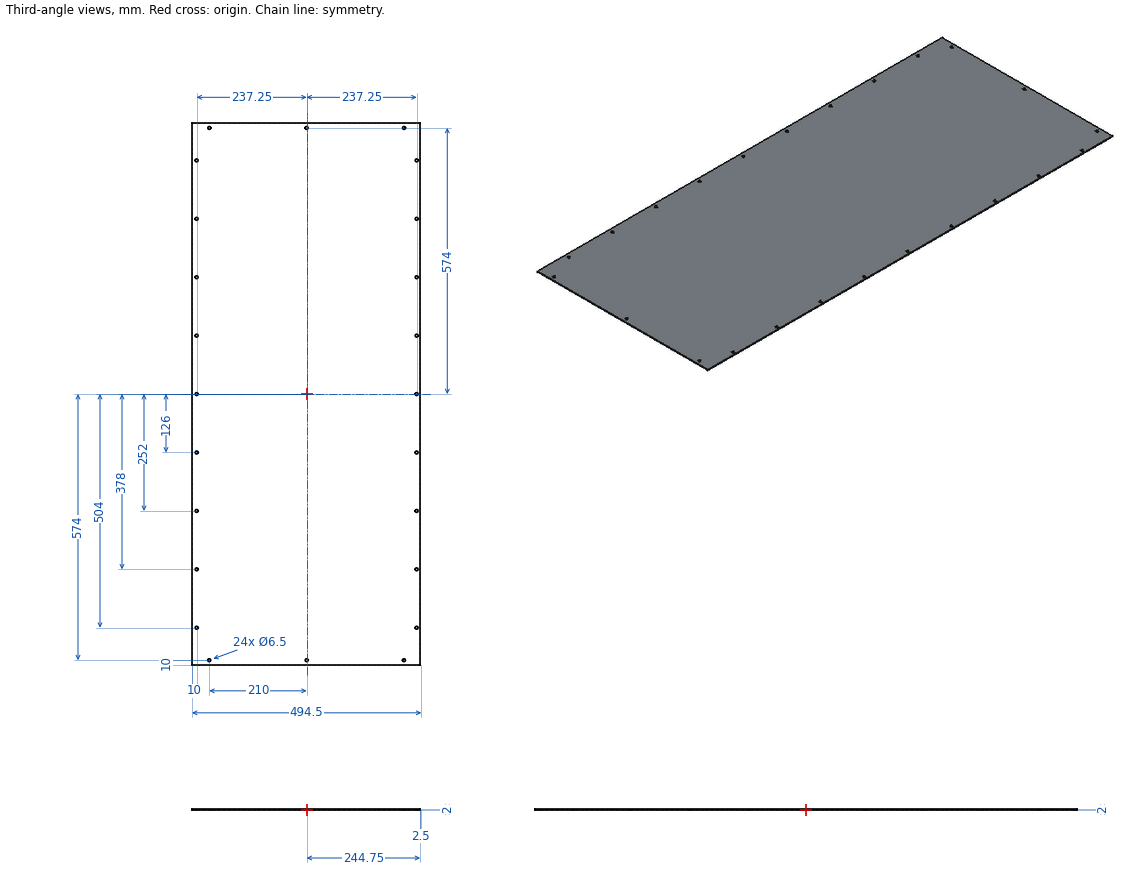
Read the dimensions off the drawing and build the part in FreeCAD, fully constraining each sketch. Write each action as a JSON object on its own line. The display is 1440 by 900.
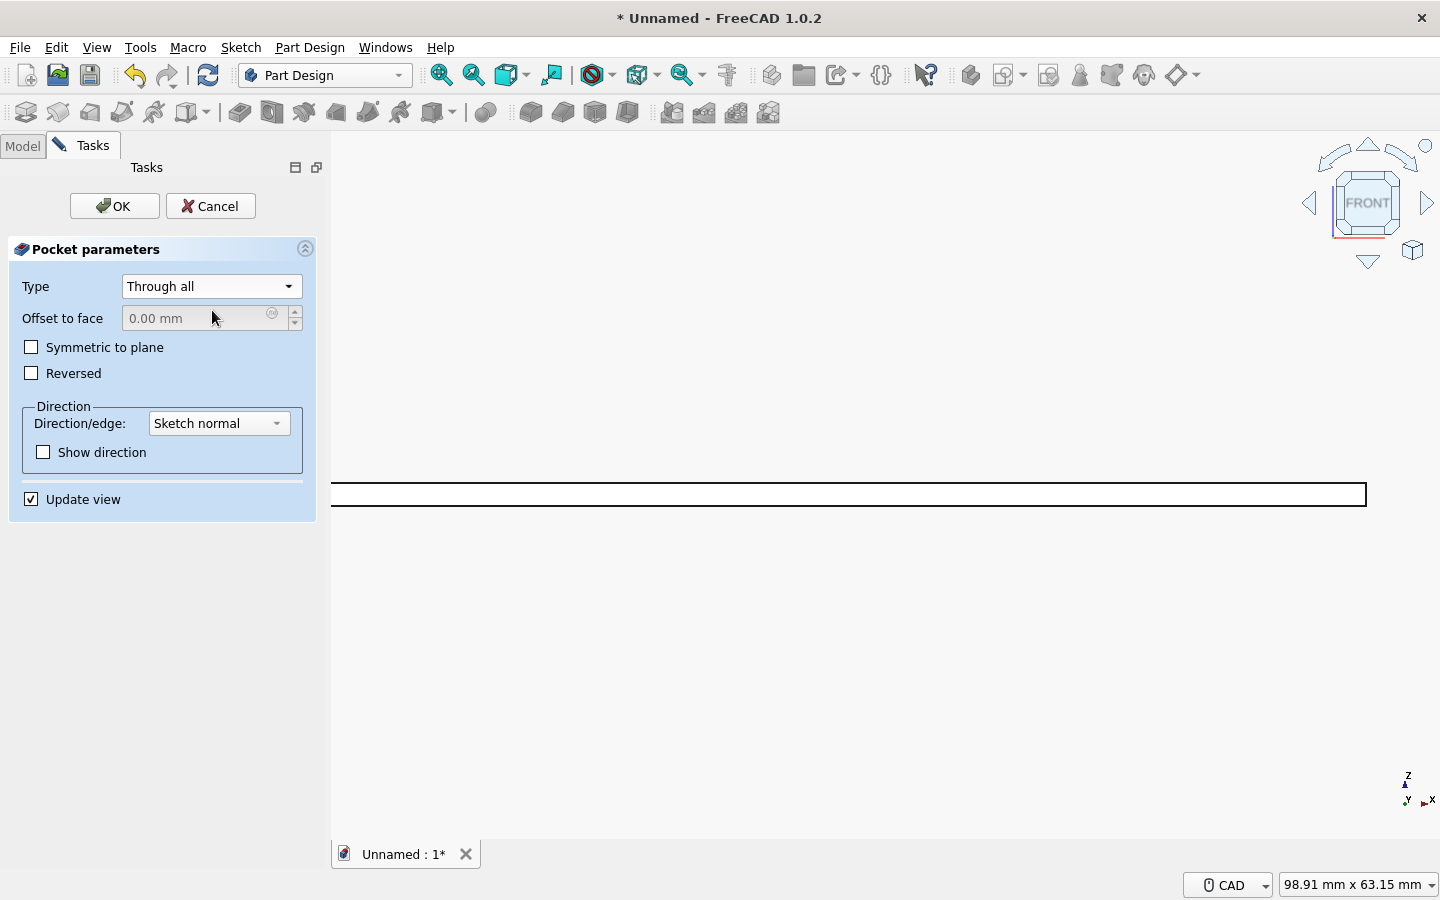
{"action": "left_click", "coordinate": [115, 206]}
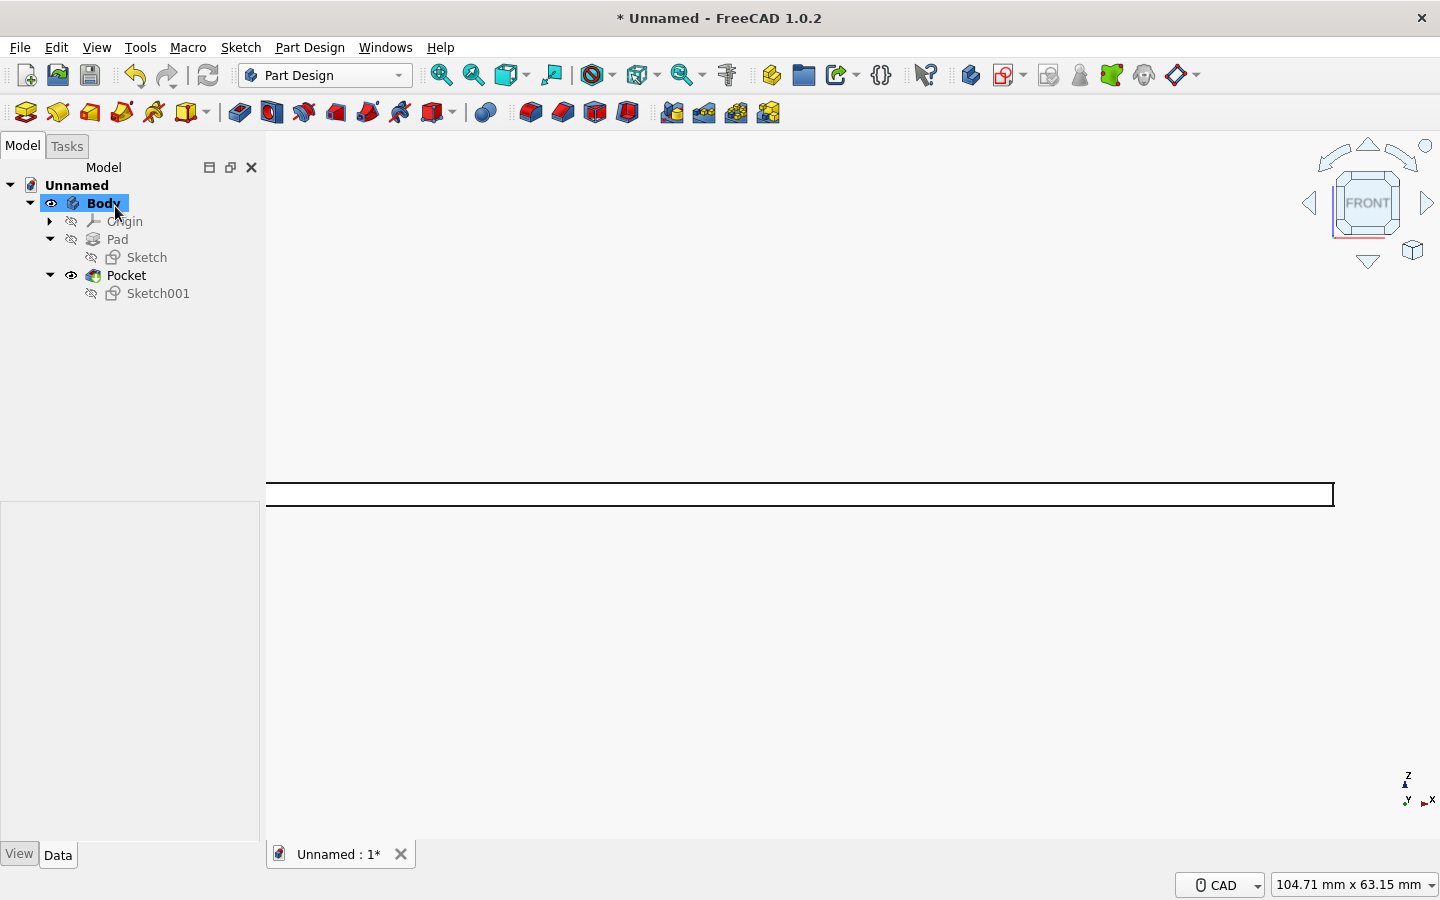
{"action": "key", "text": "0"}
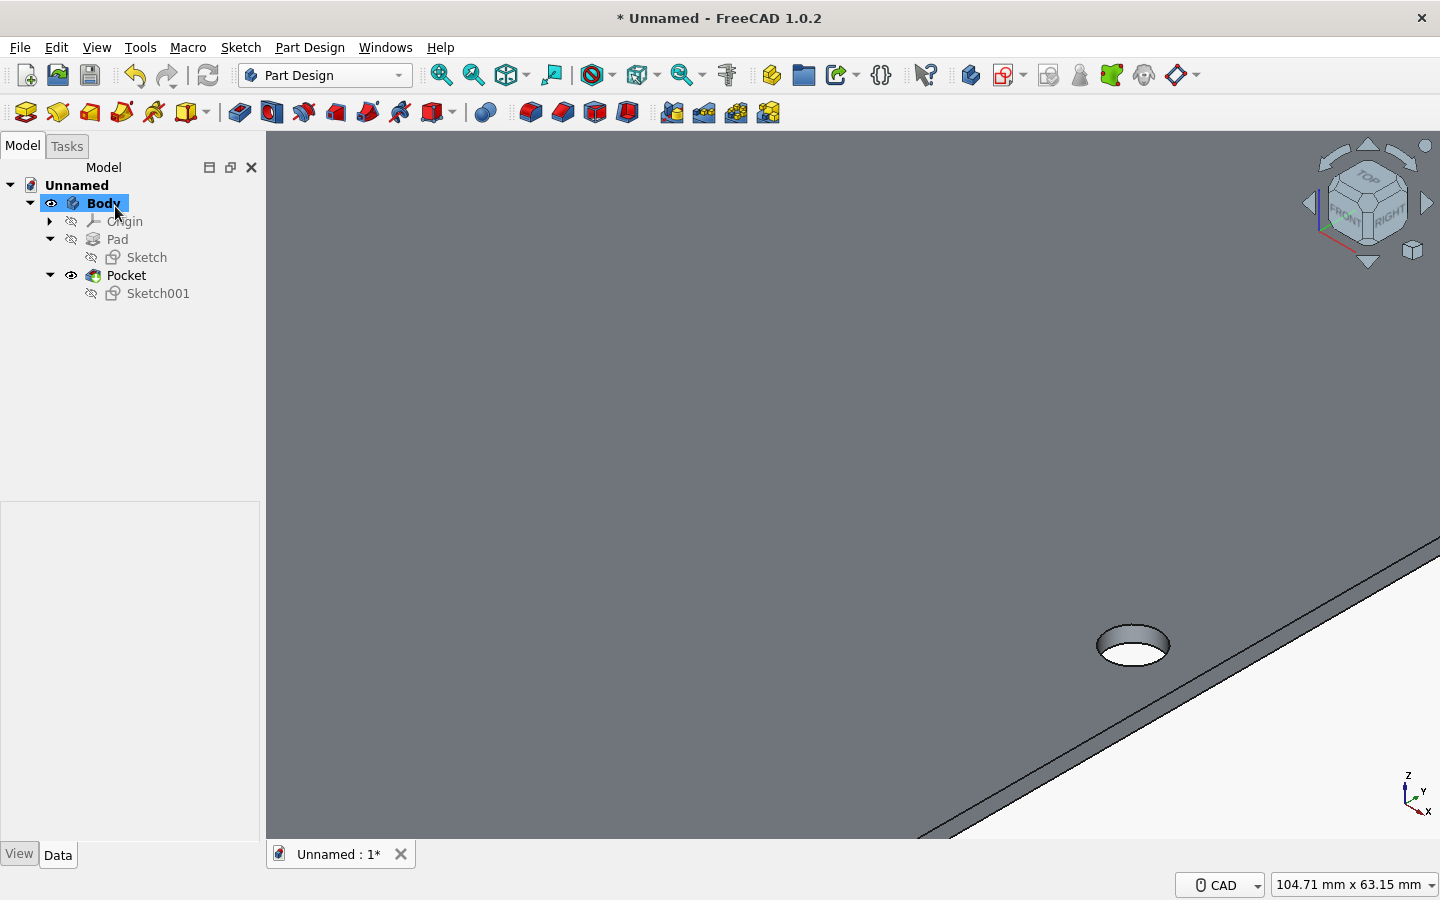
{"action": "key", "text": "v f"}